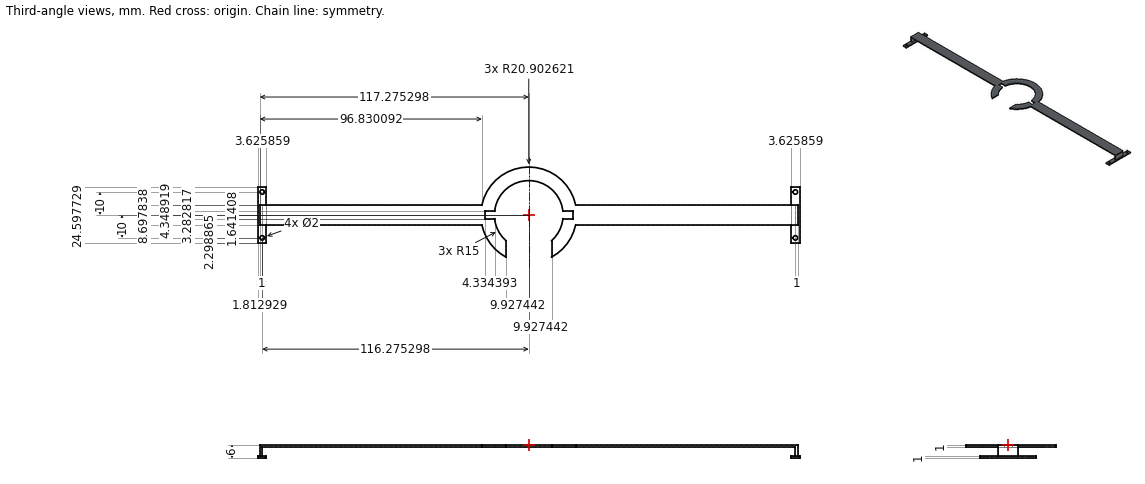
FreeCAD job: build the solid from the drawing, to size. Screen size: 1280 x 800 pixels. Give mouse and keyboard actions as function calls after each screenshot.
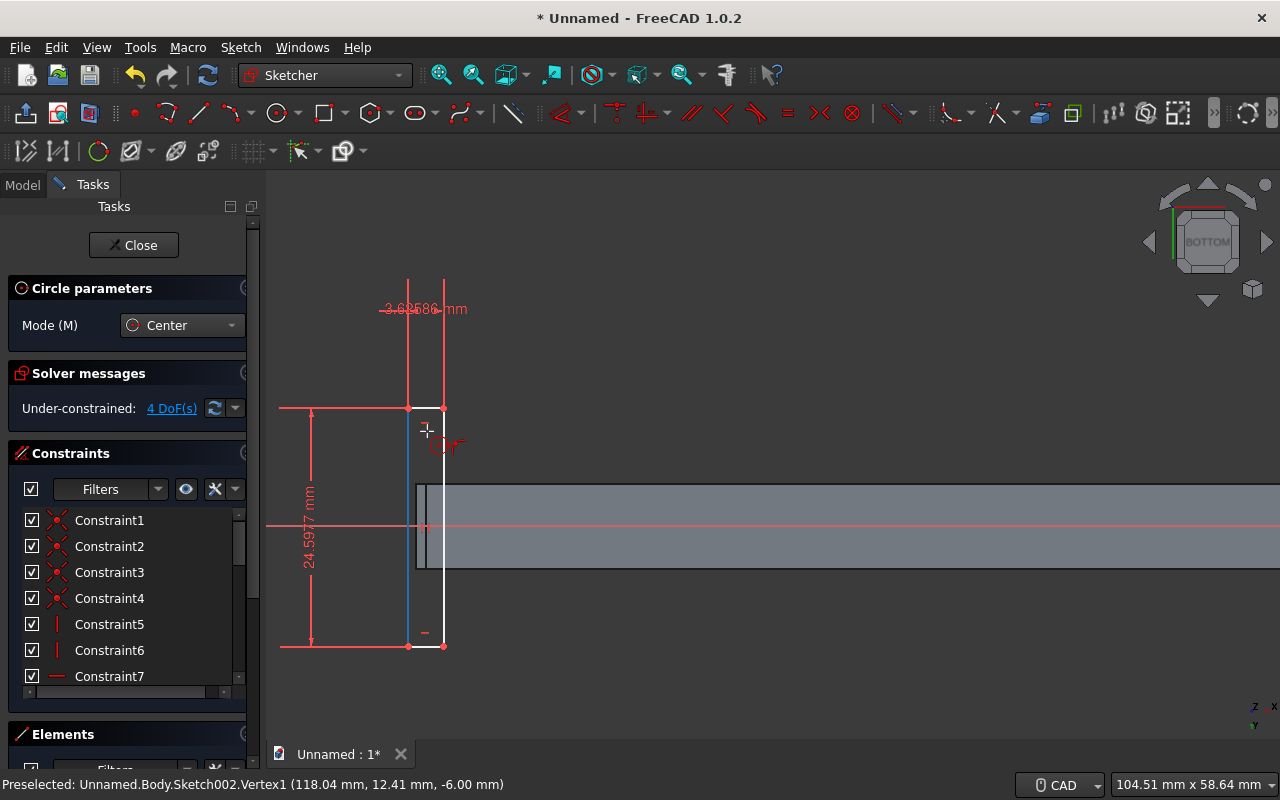
click(426, 429)
move(422, 438)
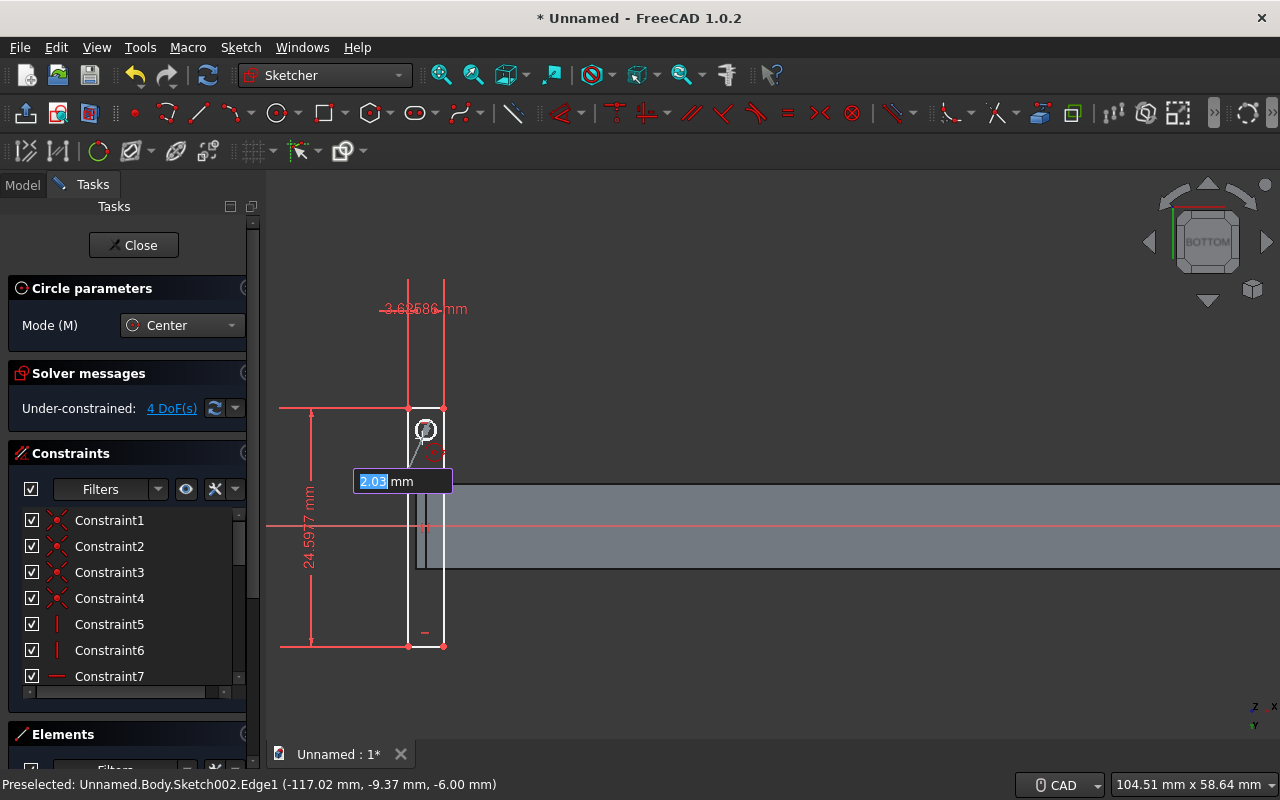
text(2)
key(Return)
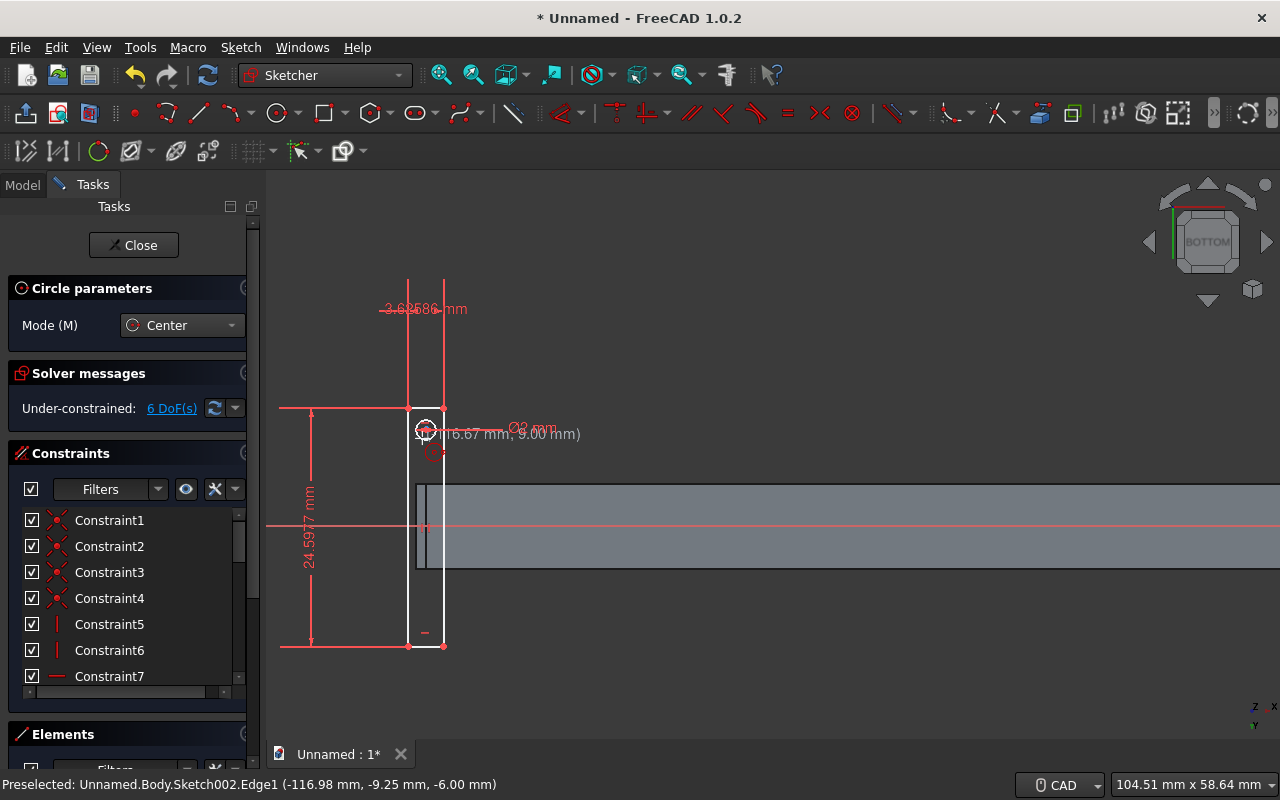
scroll(426, 623, up, 5)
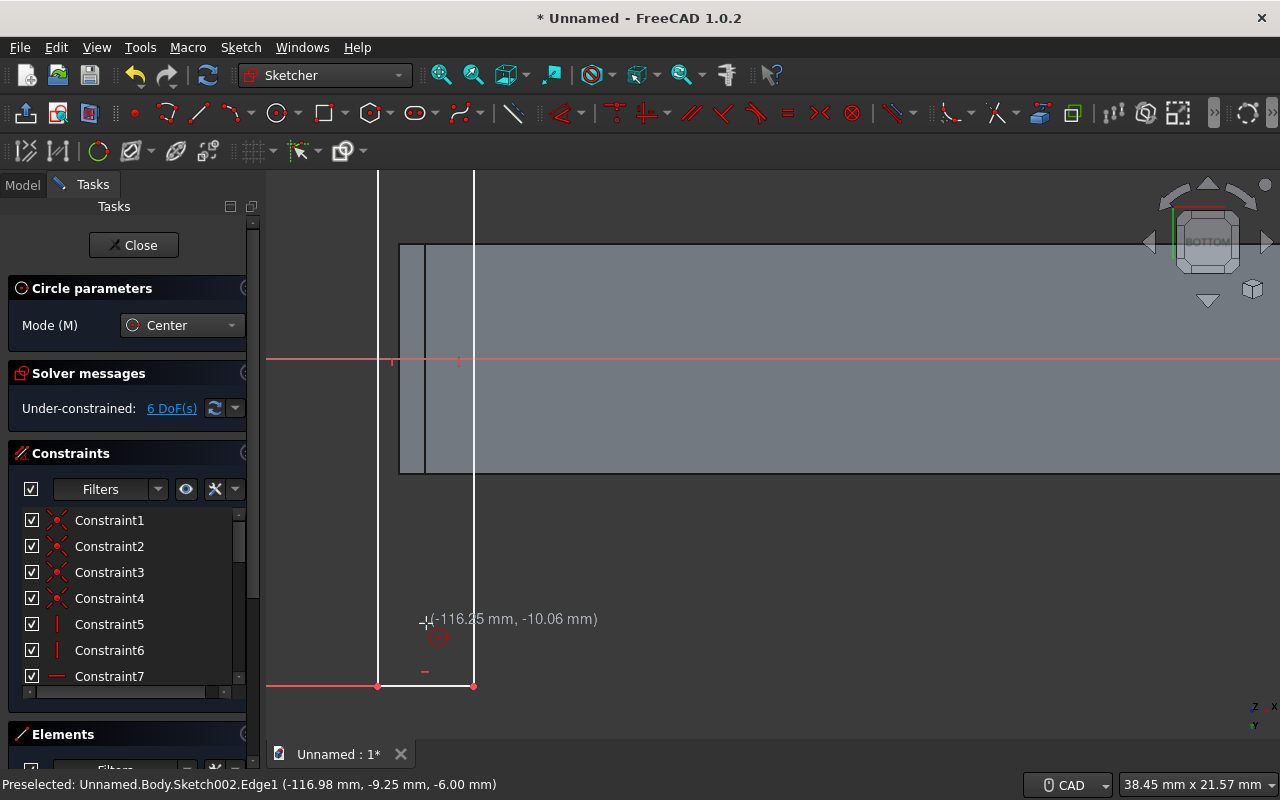
scroll(426, 464, down, 12)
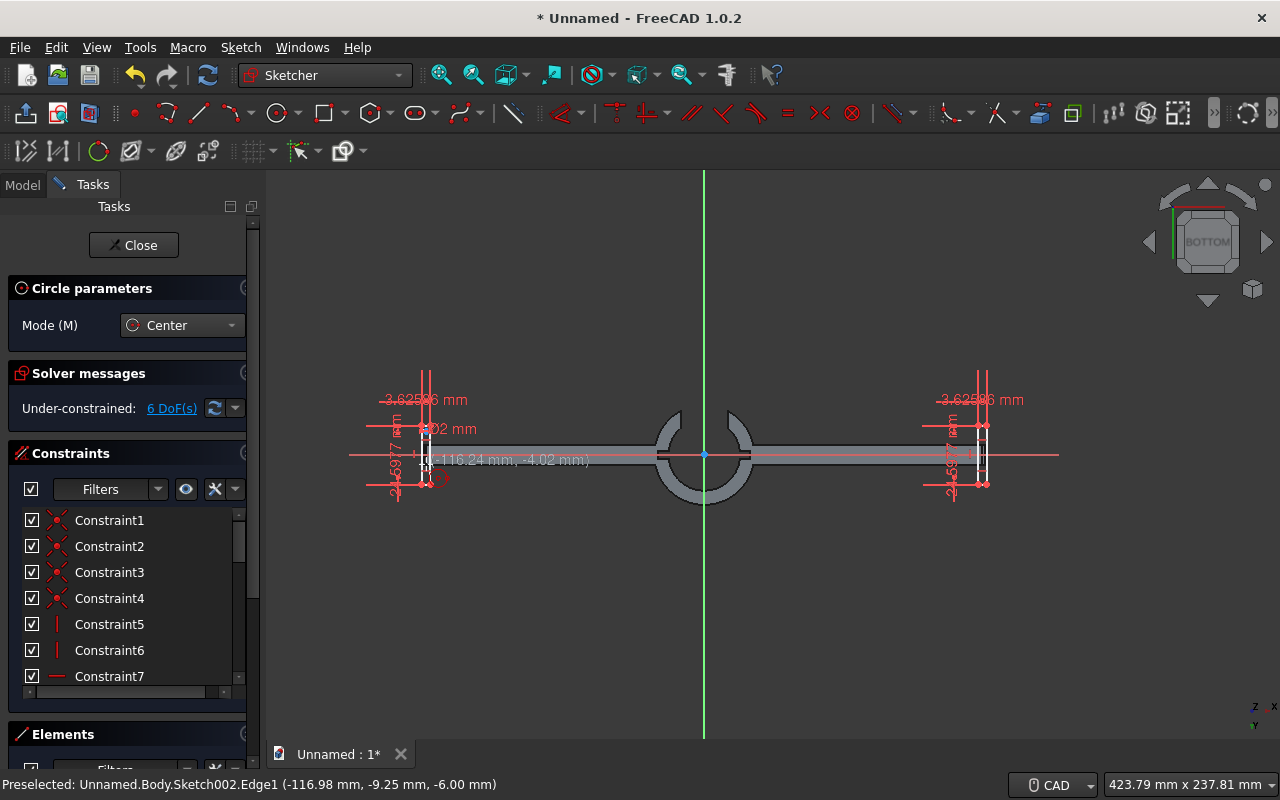
scroll(426, 479, up, 7)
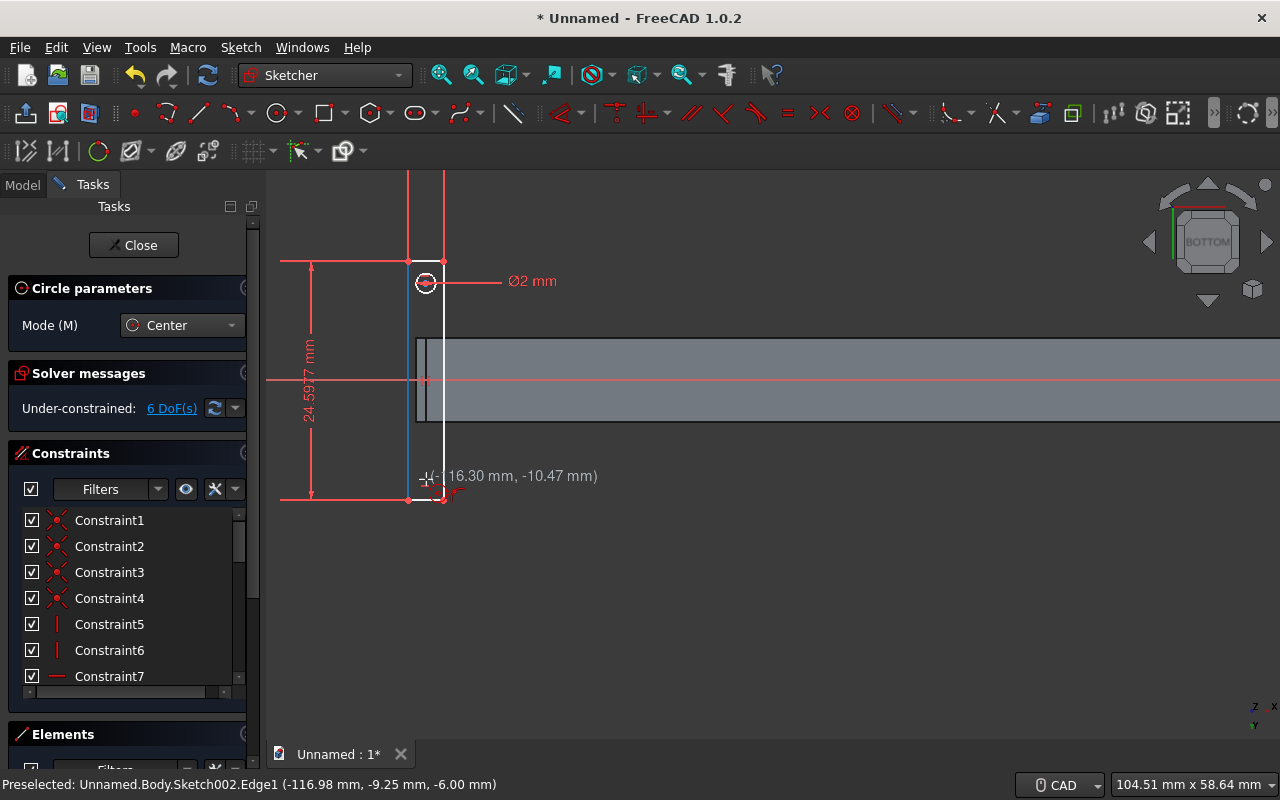
click(426, 477)
move(429, 468)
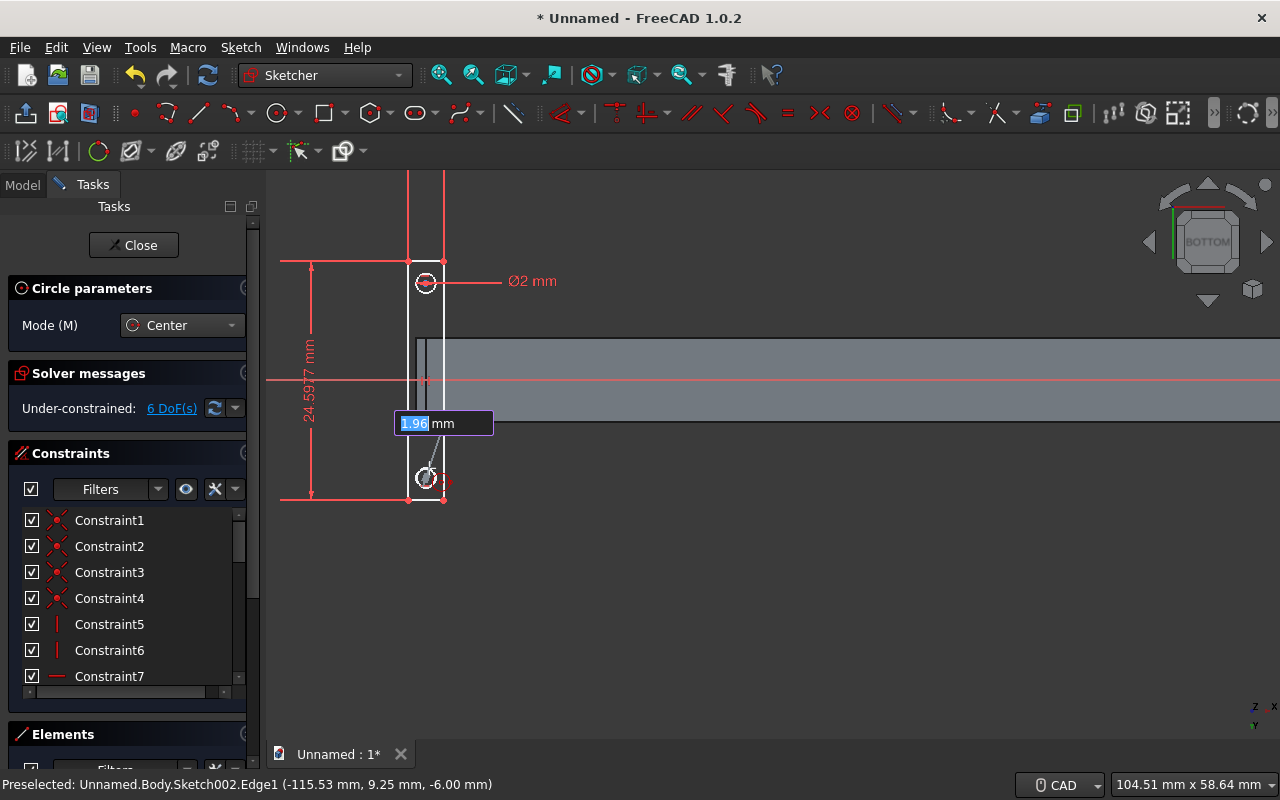
text(2)
key(Return)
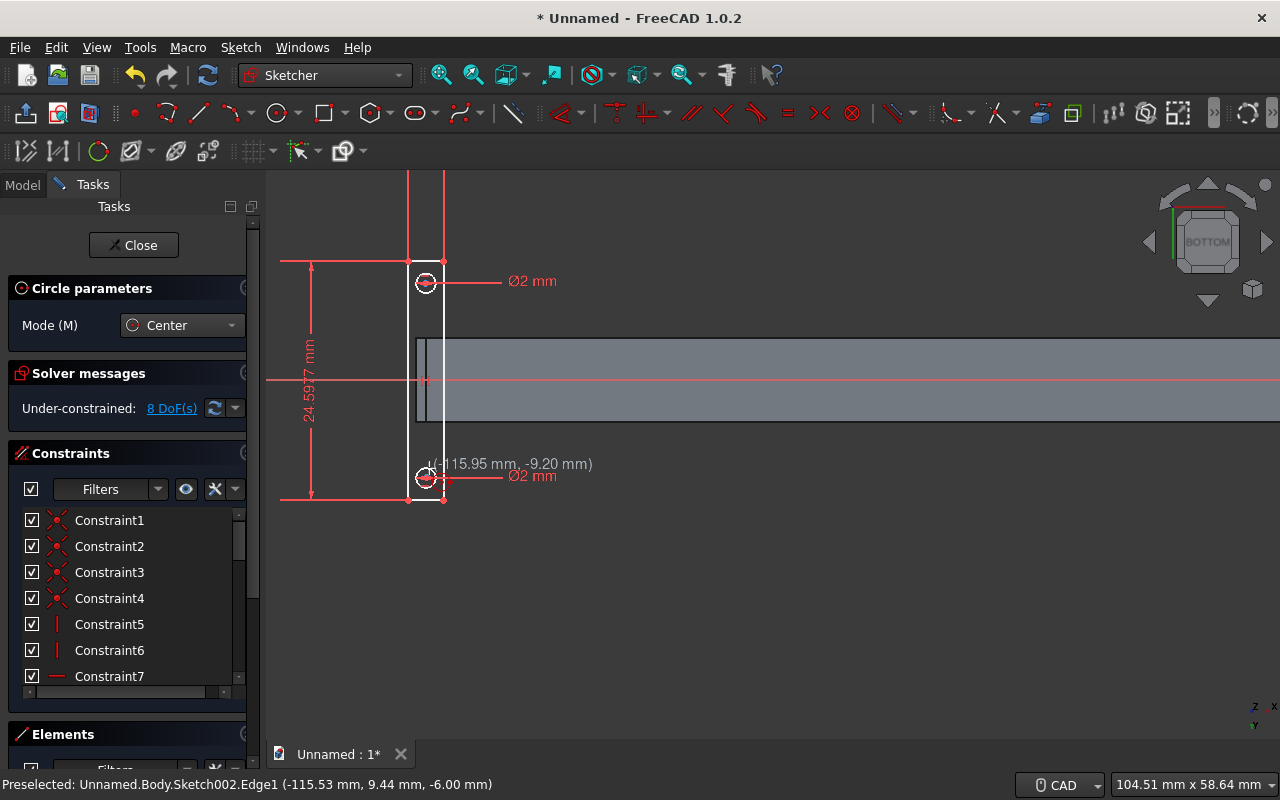
scroll(426, 479, down, 7)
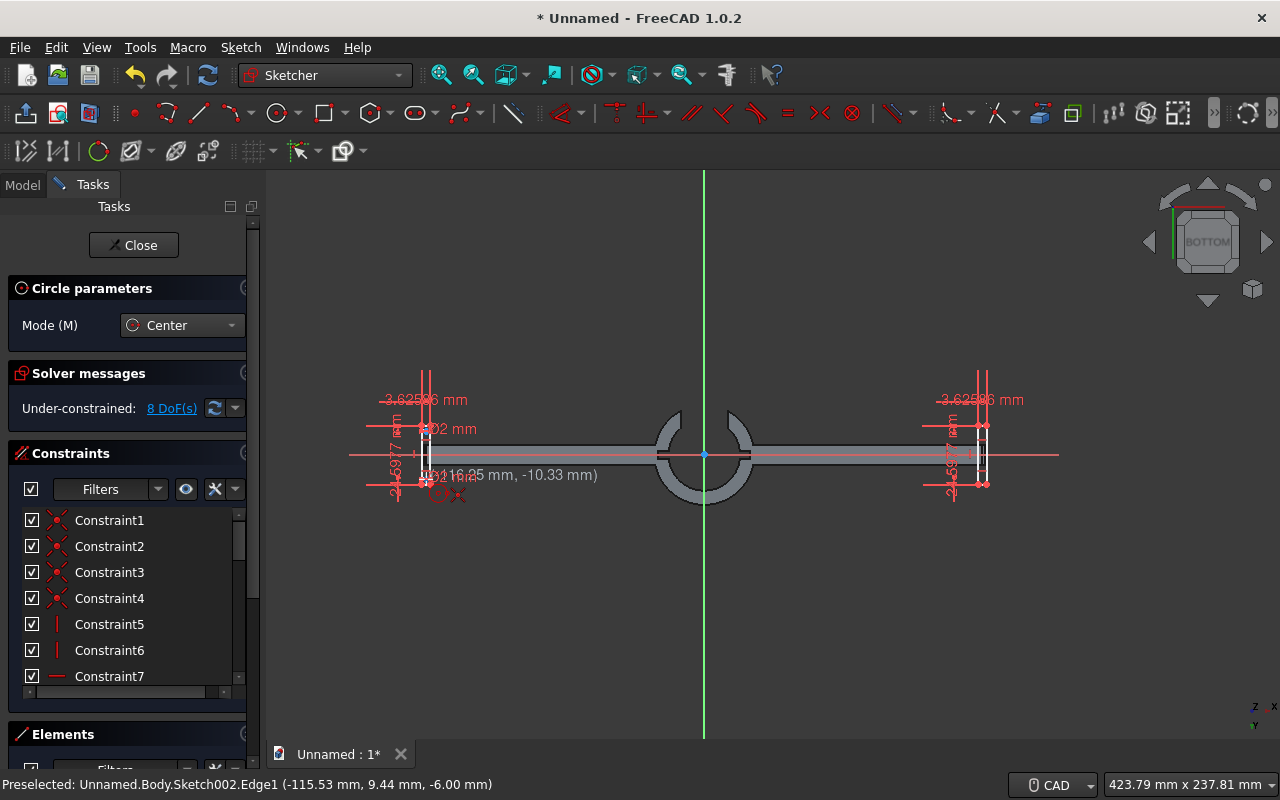
scroll(982, 431, up, 12)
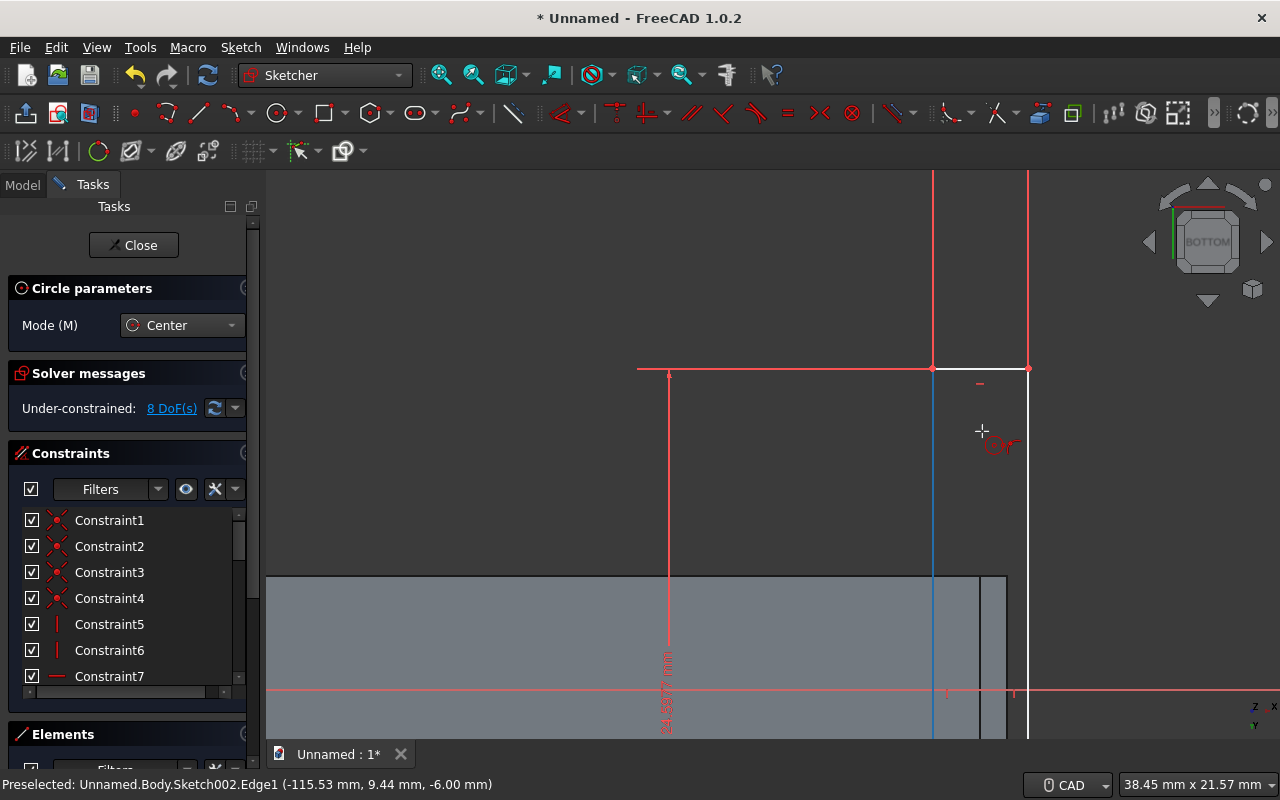
scroll(983, 431, down, 12)